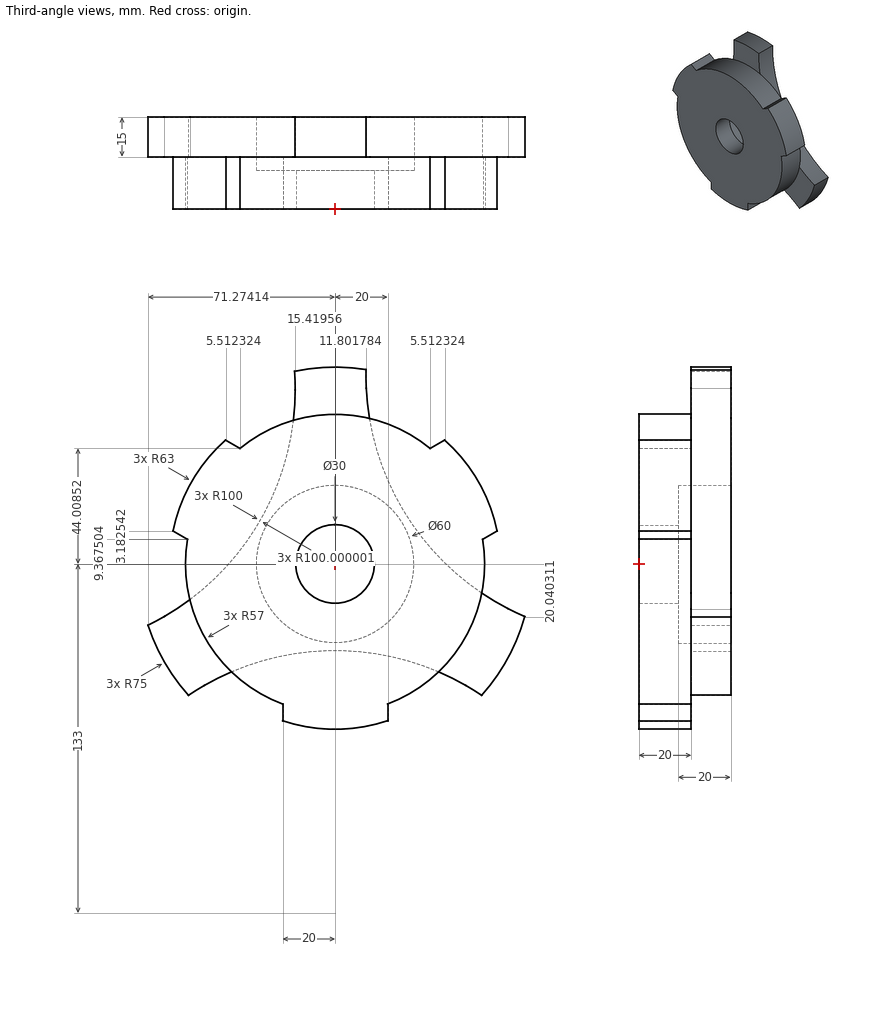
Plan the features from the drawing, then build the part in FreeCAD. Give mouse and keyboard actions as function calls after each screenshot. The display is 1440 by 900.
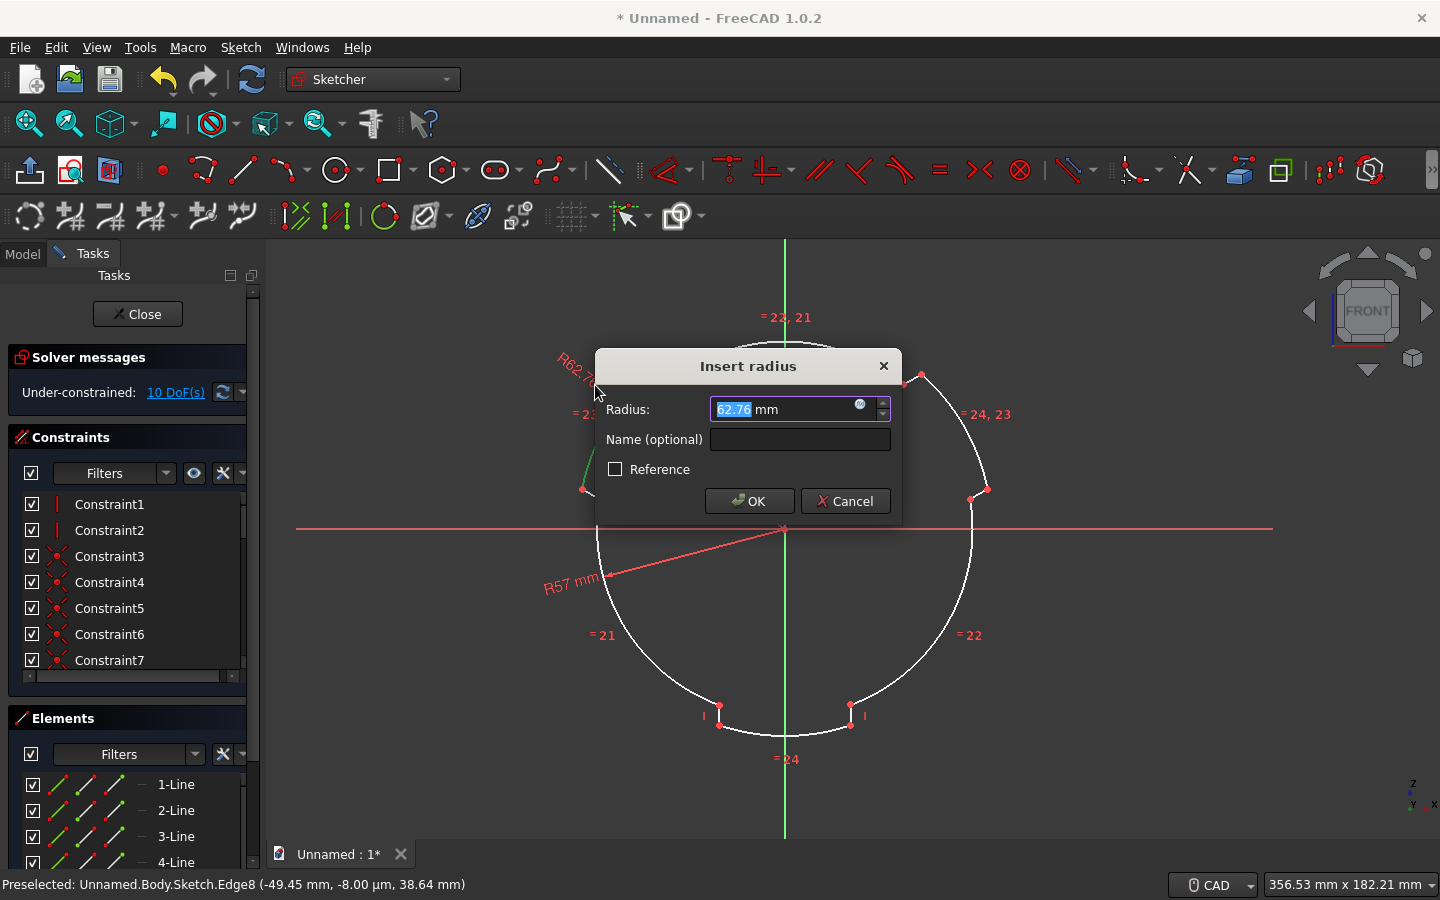
text(63)
key(Return)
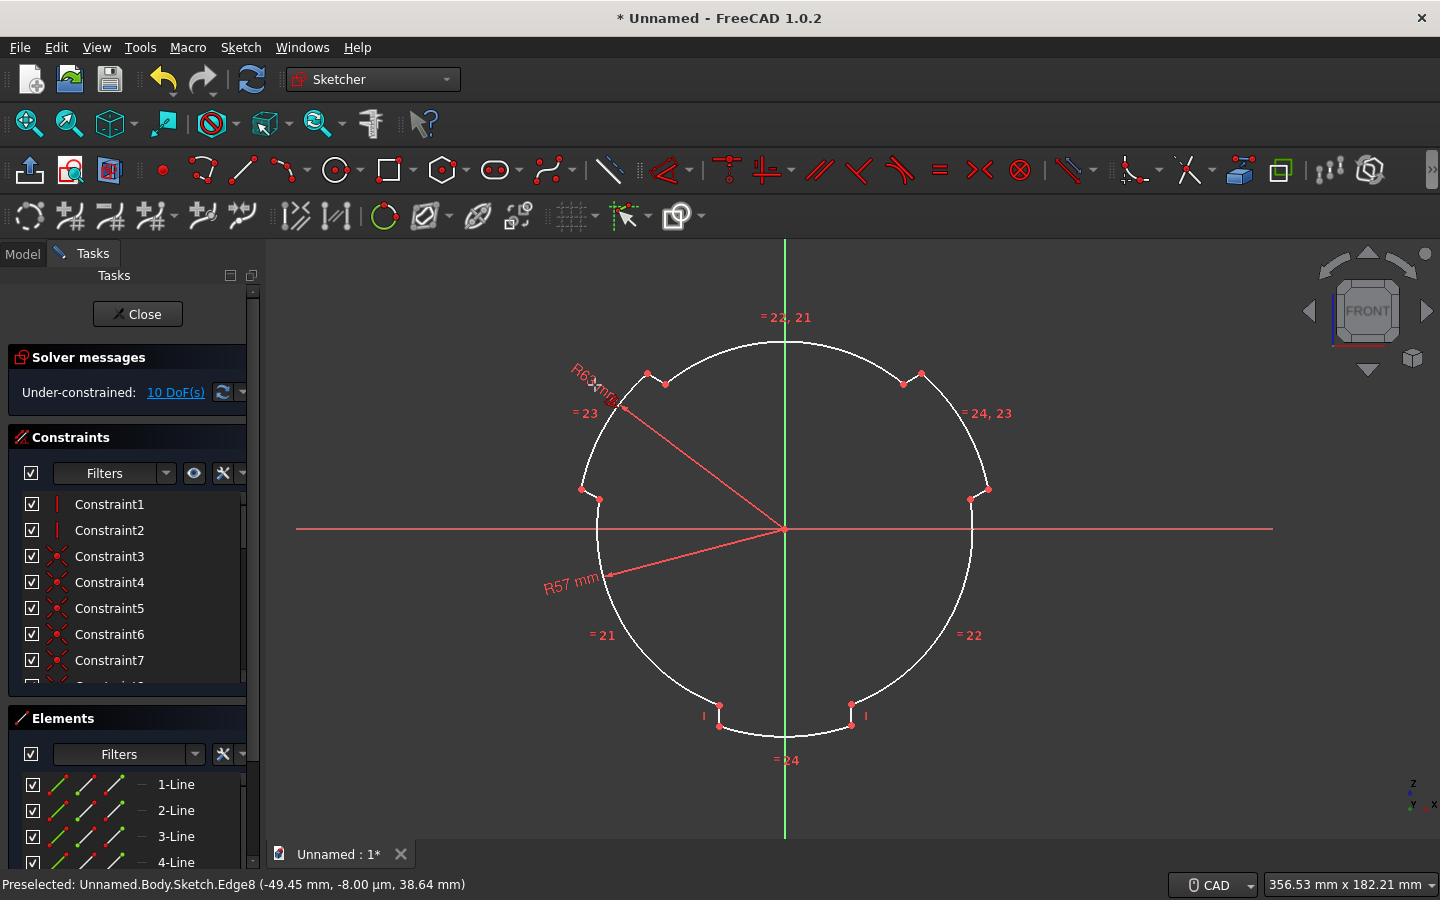
click(719, 726)
click(752, 760)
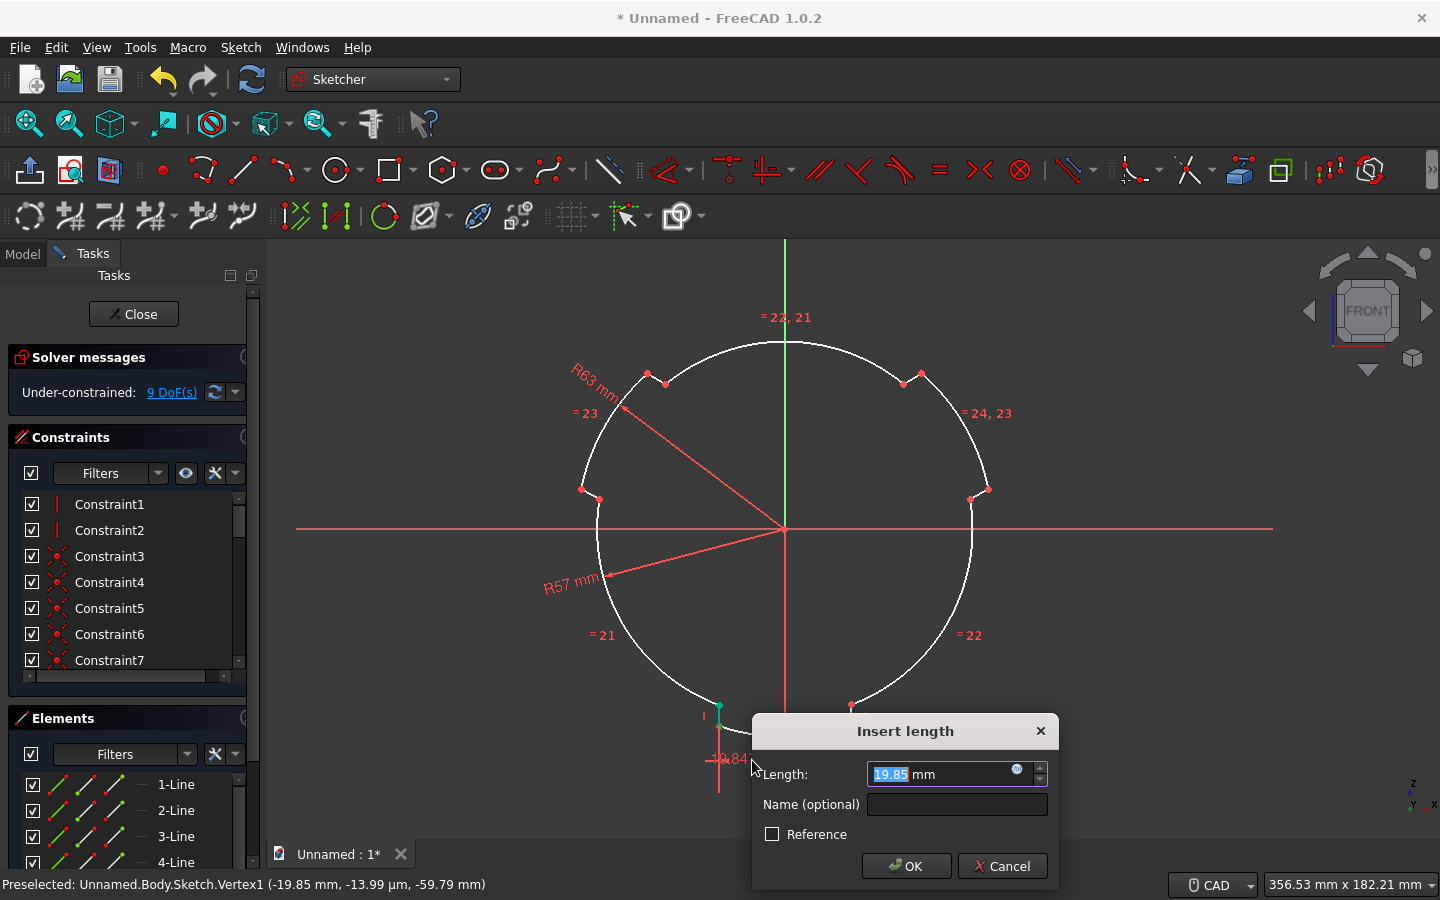
text(20)
key(Return)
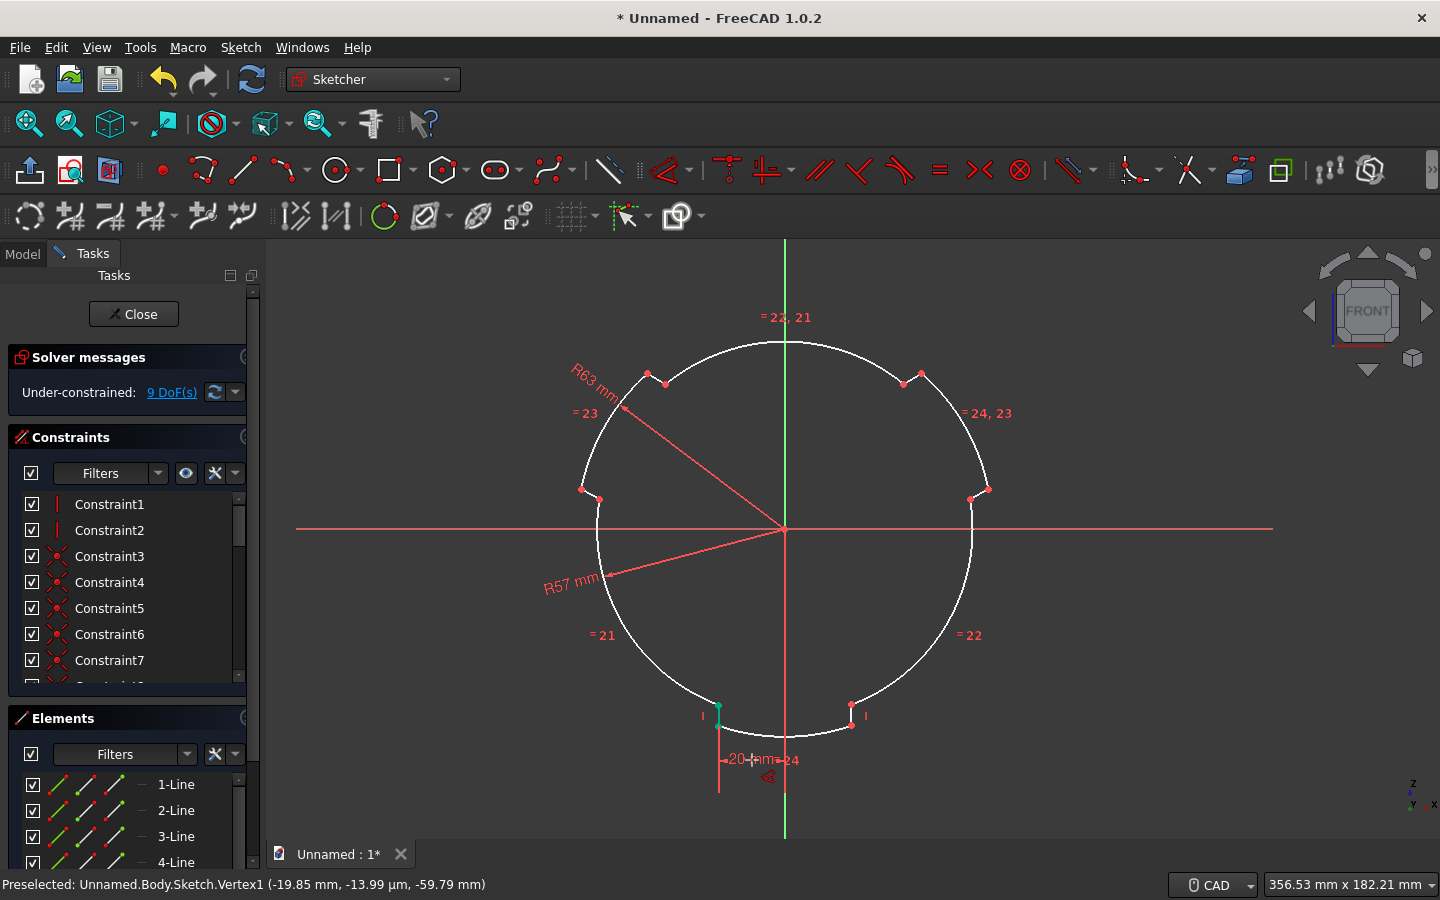
click(851, 705)
click(818, 495)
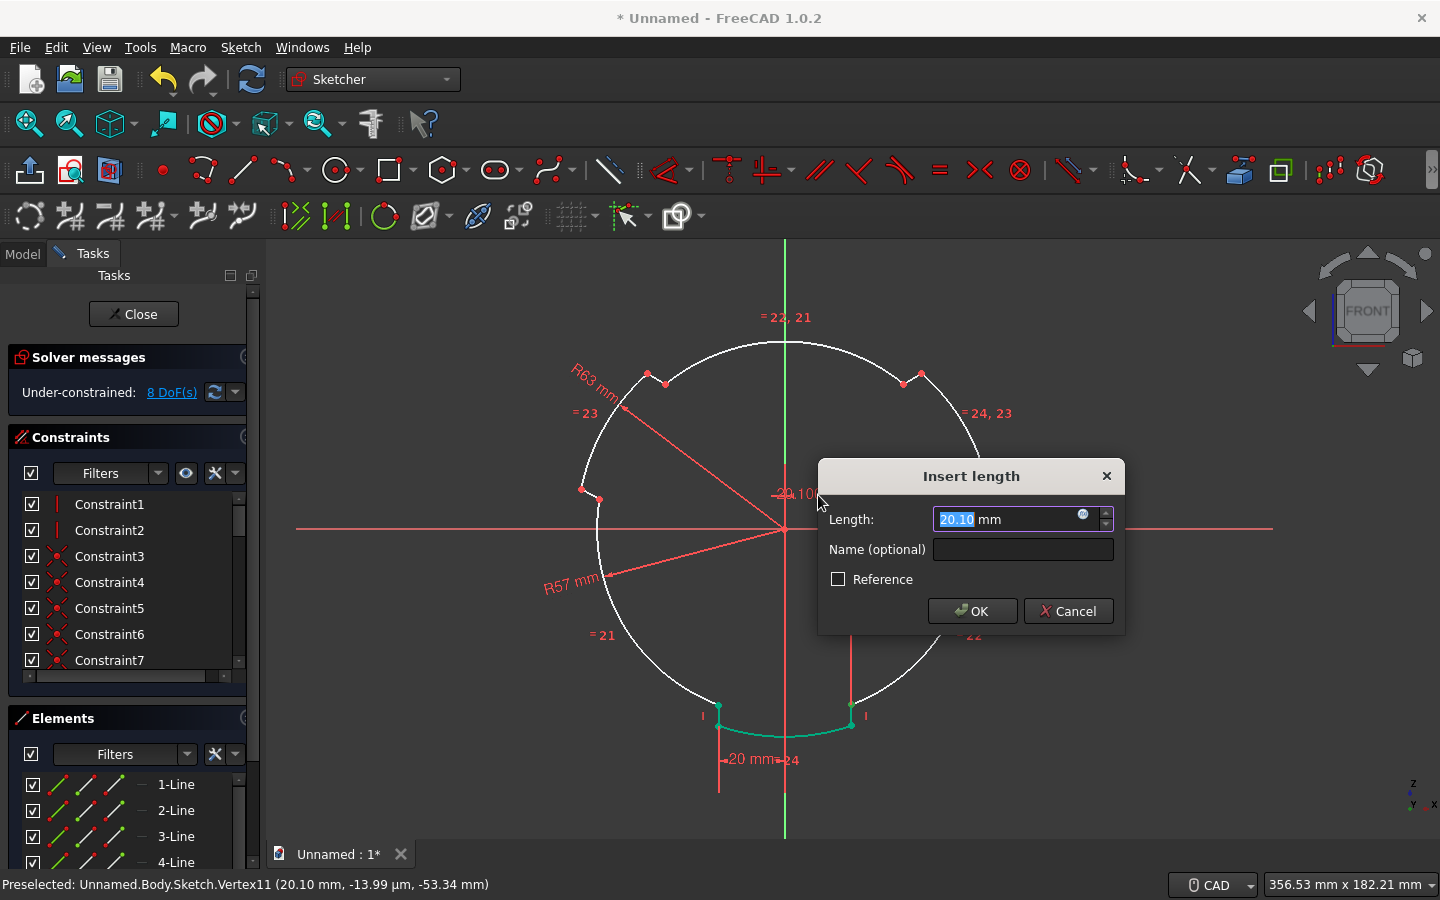
text(20)
key(Return)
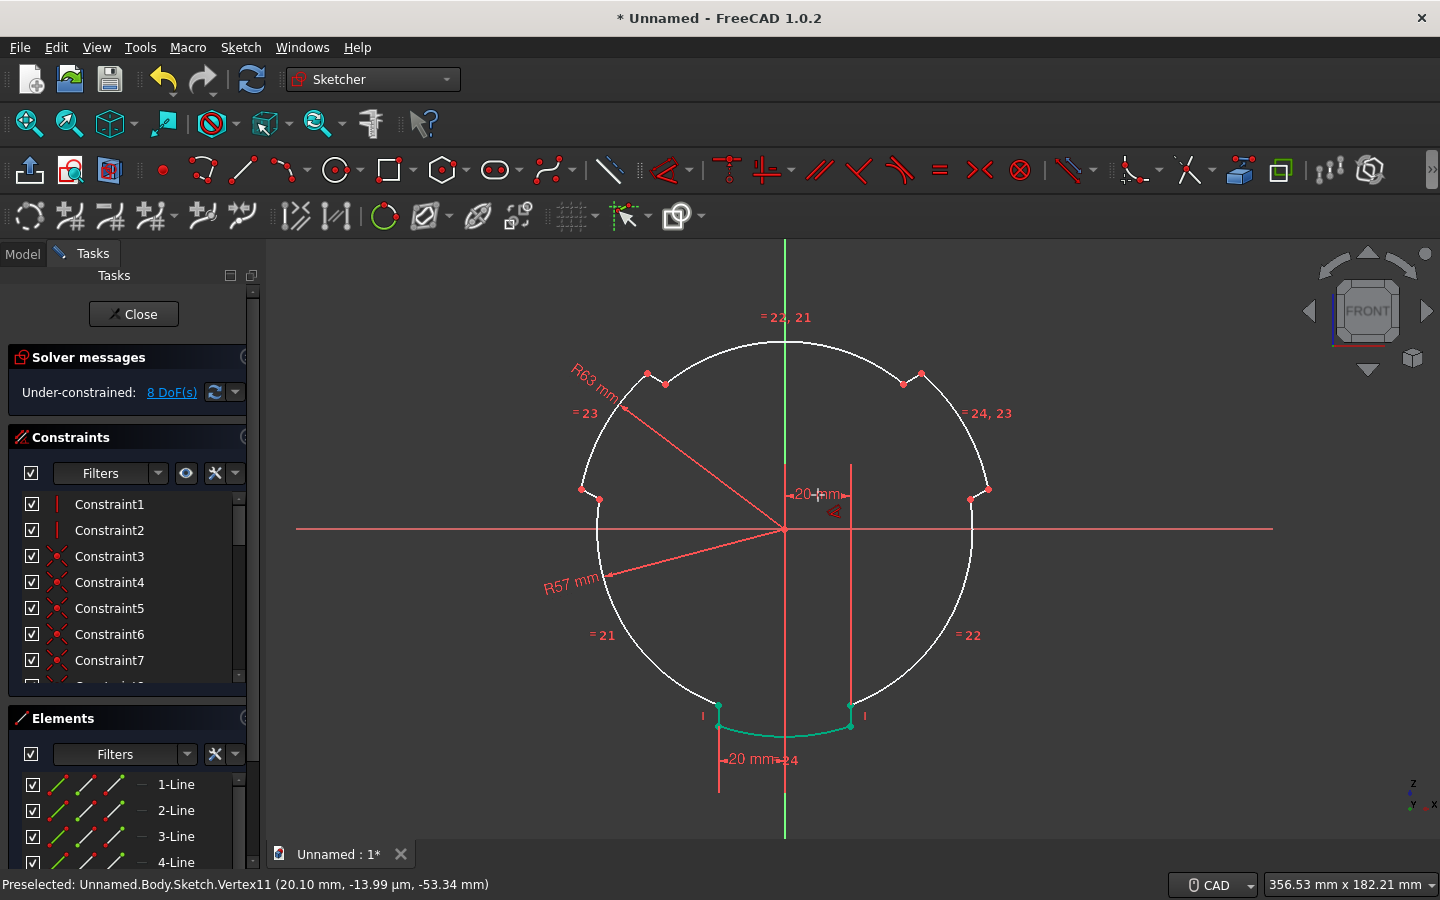
scroll(600, 499, up, 2)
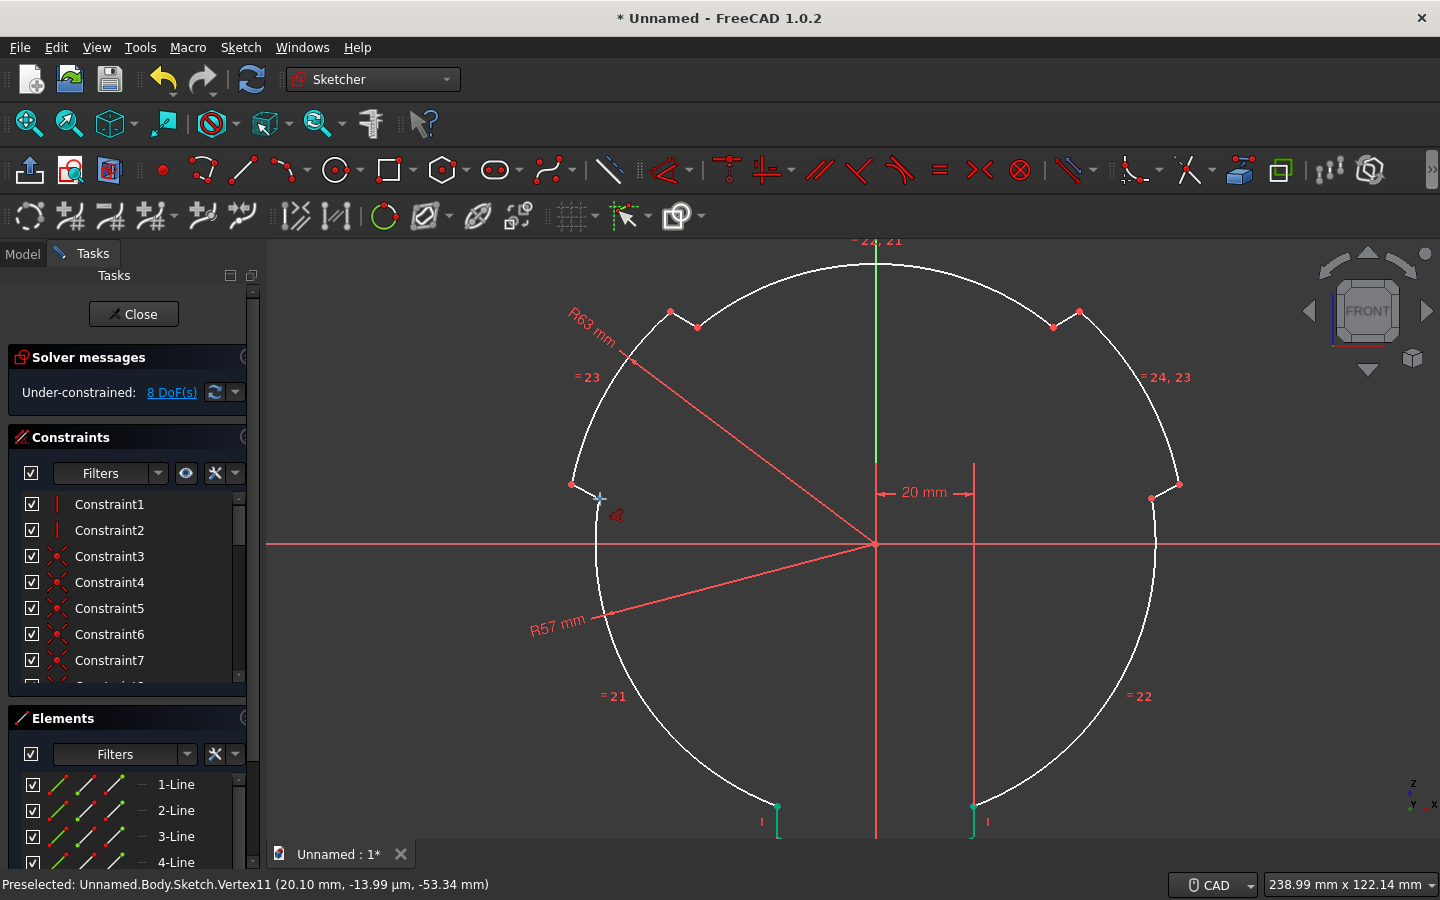
click(599, 499)
click(565, 521)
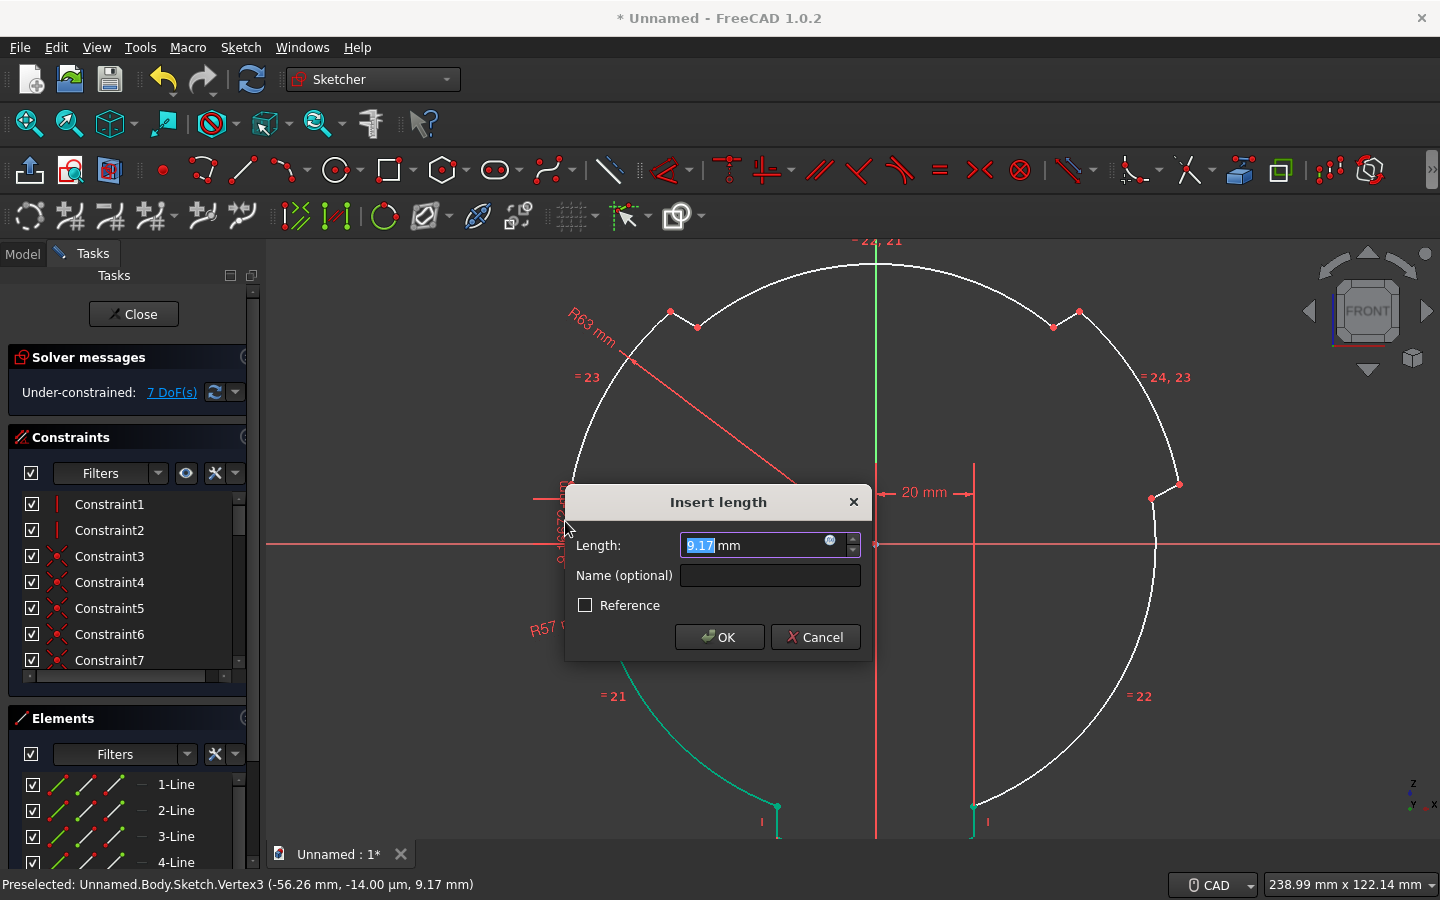
text(9.367504)
key(Return)